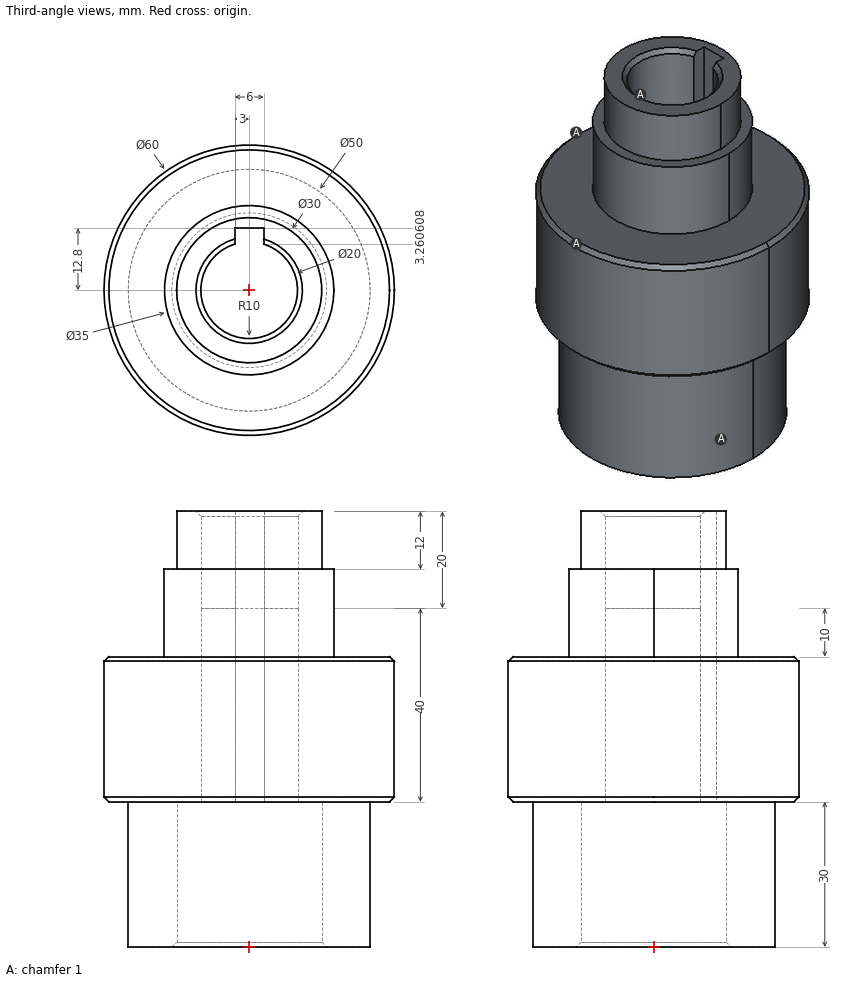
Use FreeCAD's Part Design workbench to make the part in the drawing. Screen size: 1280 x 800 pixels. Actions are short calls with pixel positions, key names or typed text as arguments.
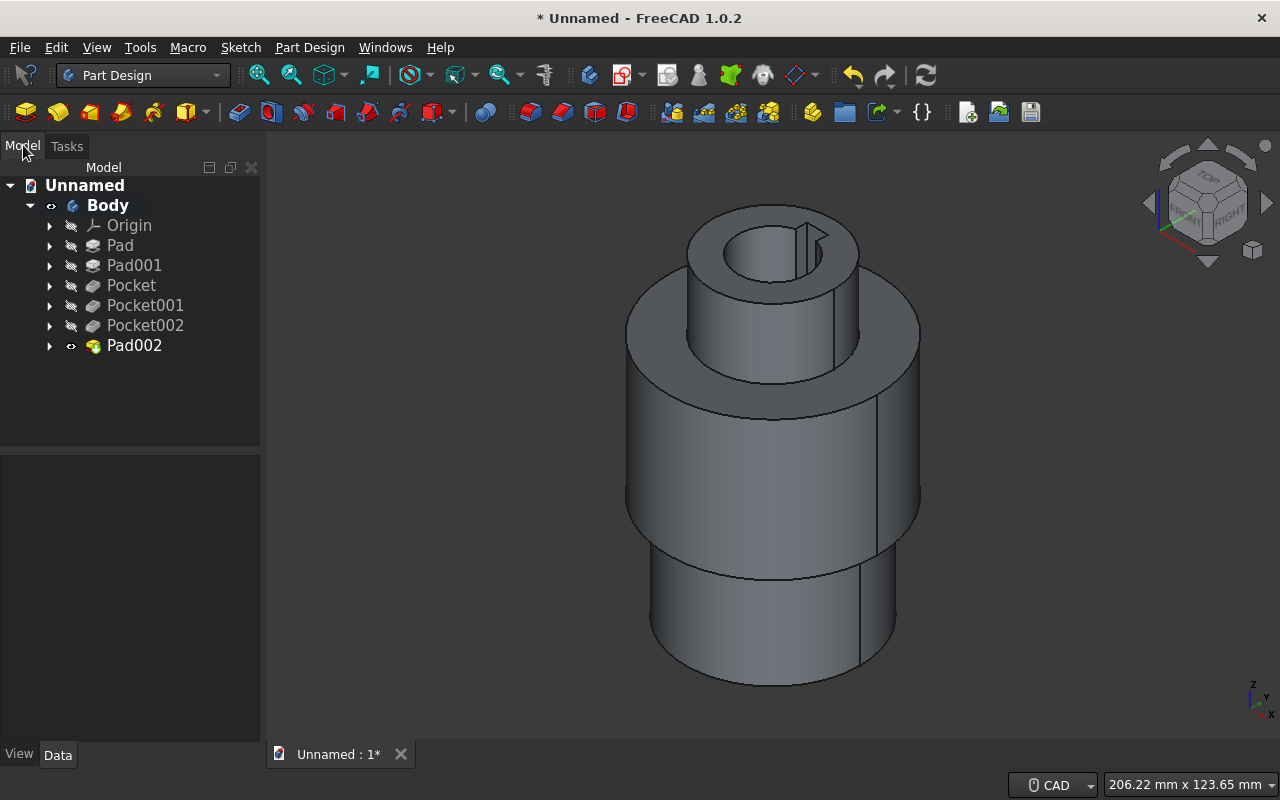
click(50, 226)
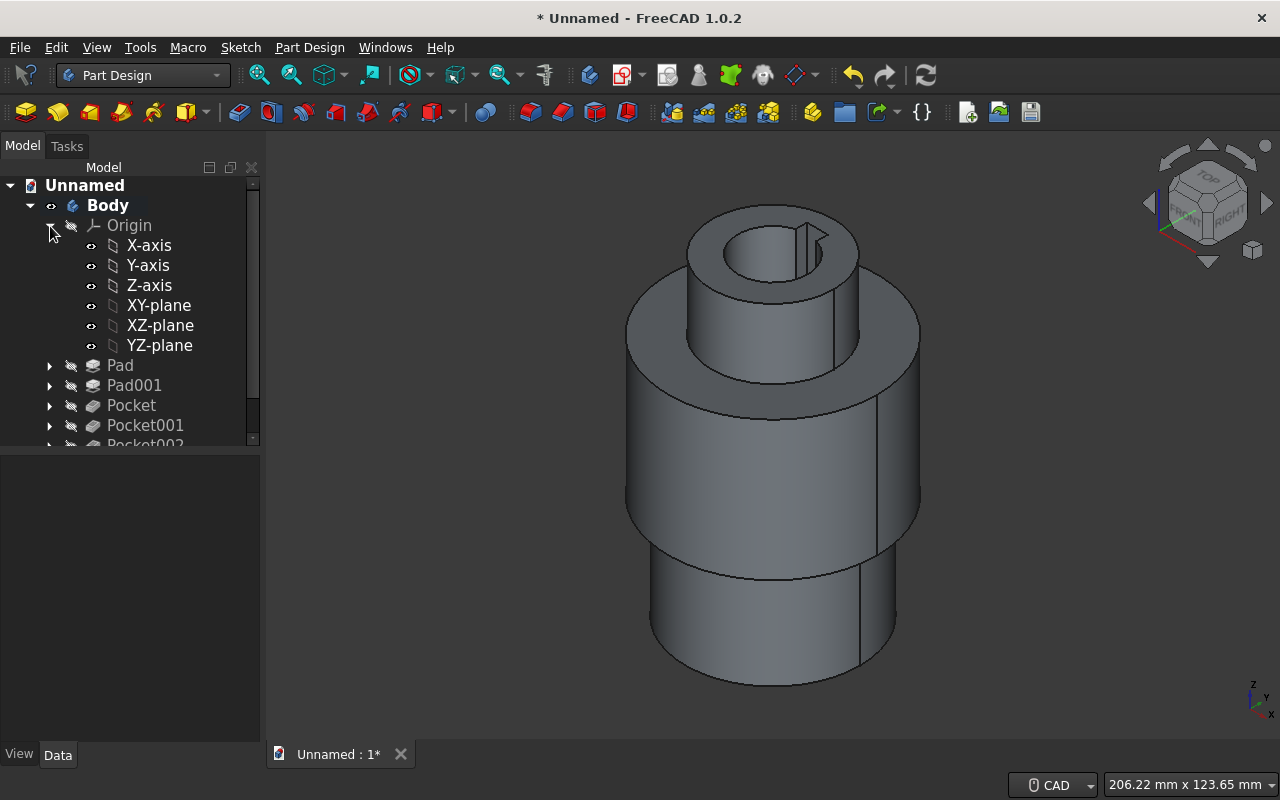
click(136, 306)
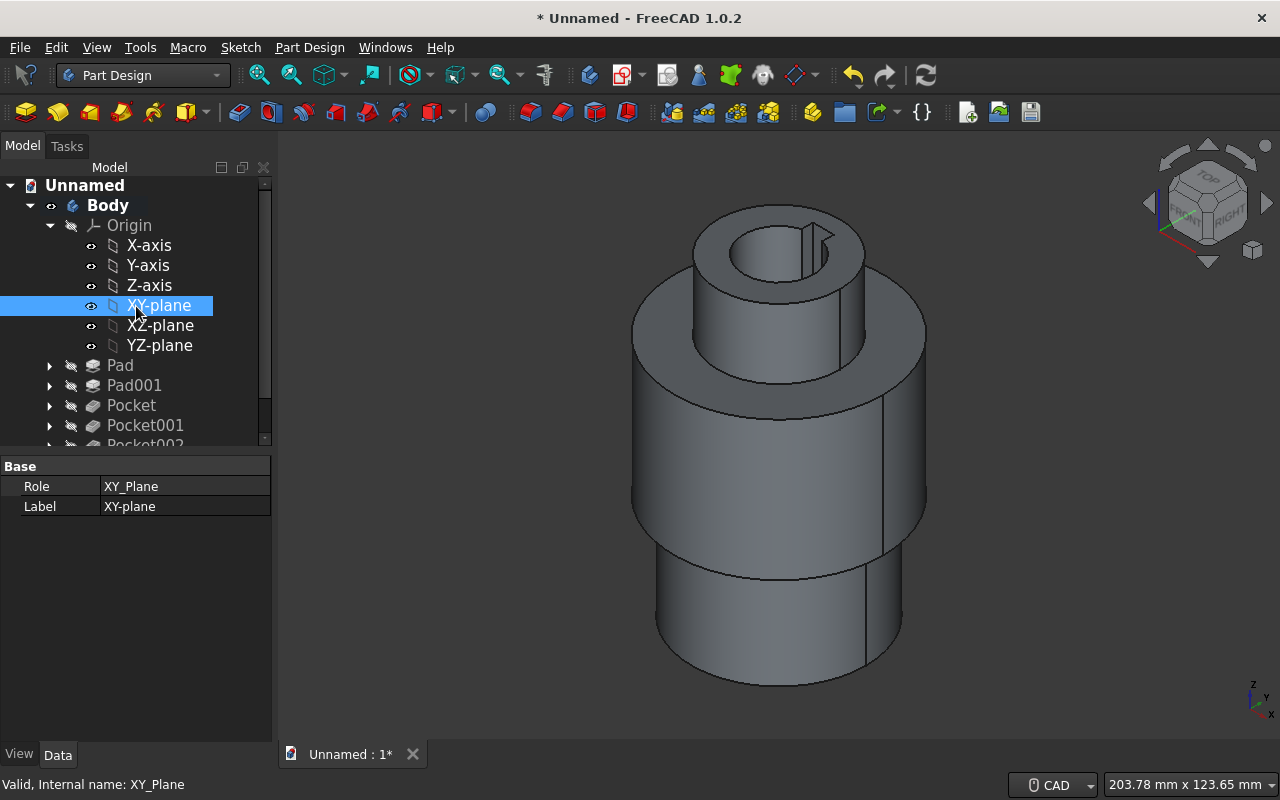
click(796, 76)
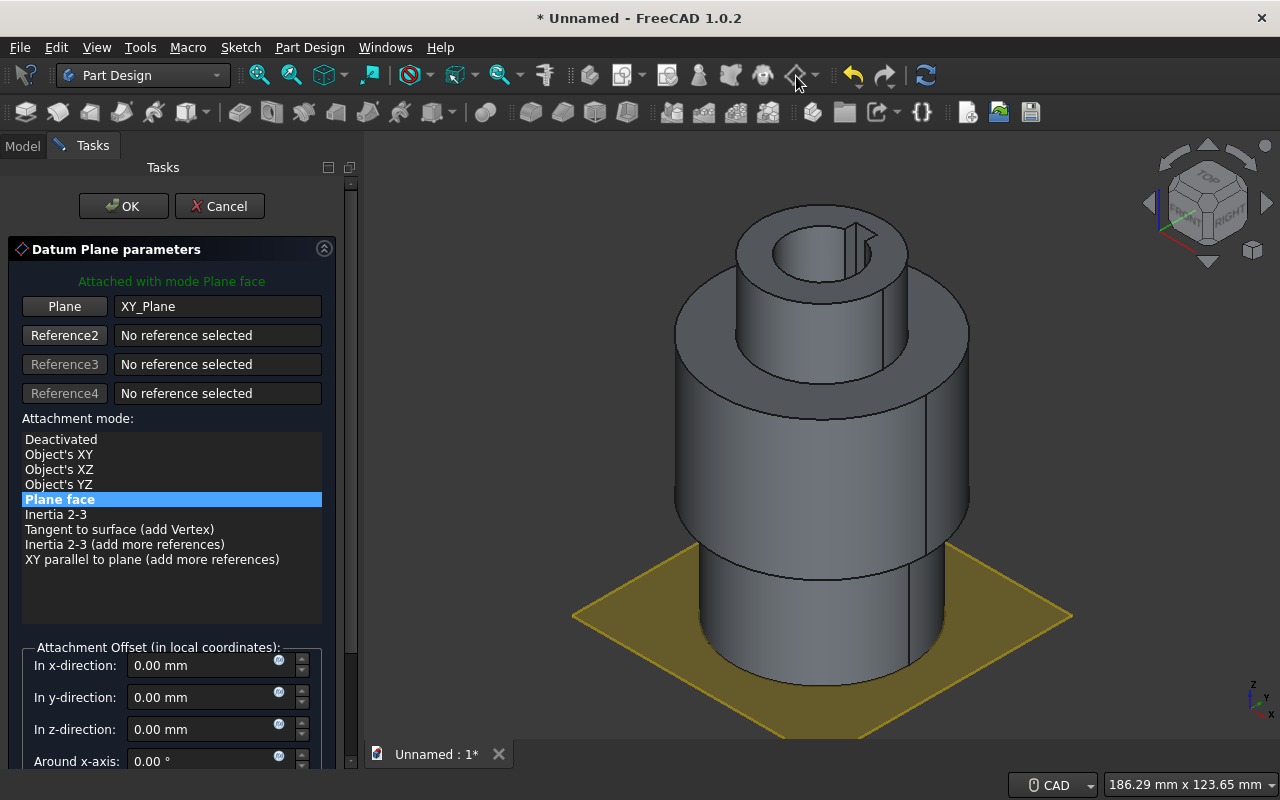
triple_click(210, 729)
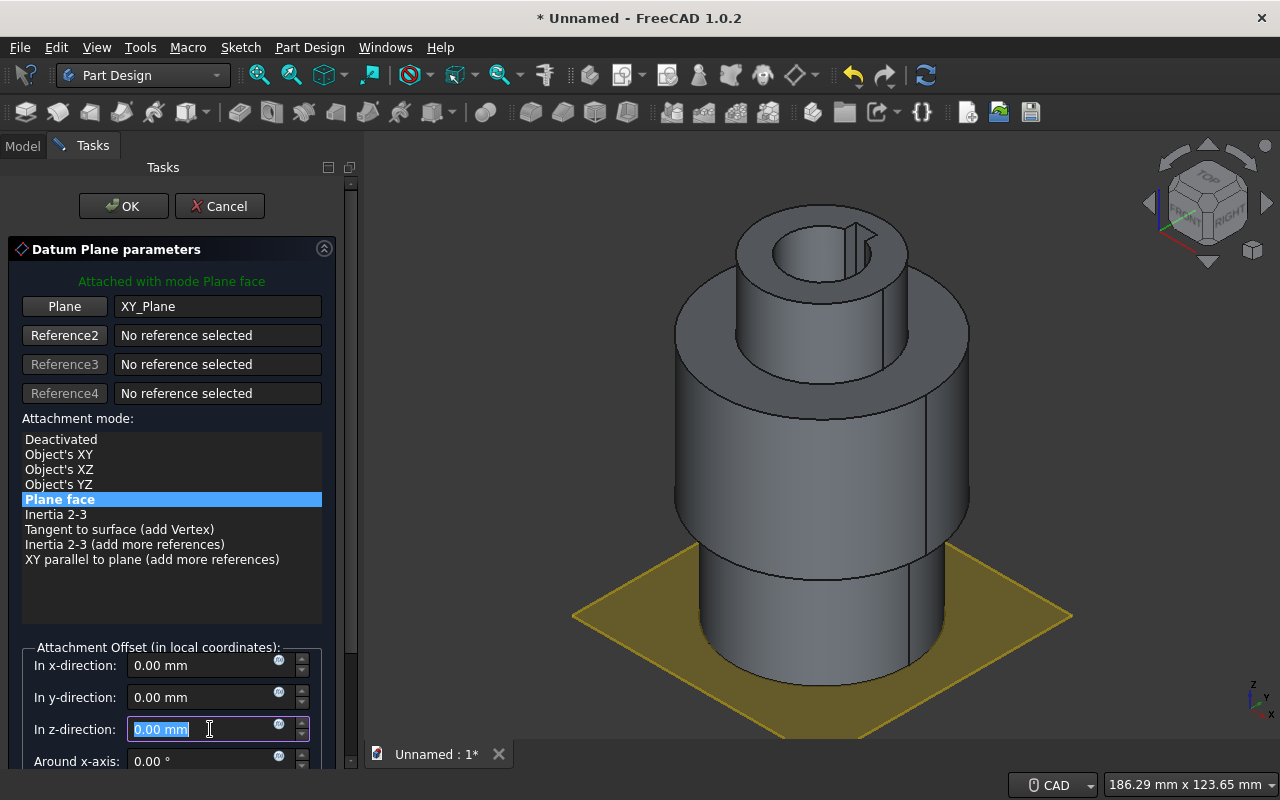
text(60)
key(Tab)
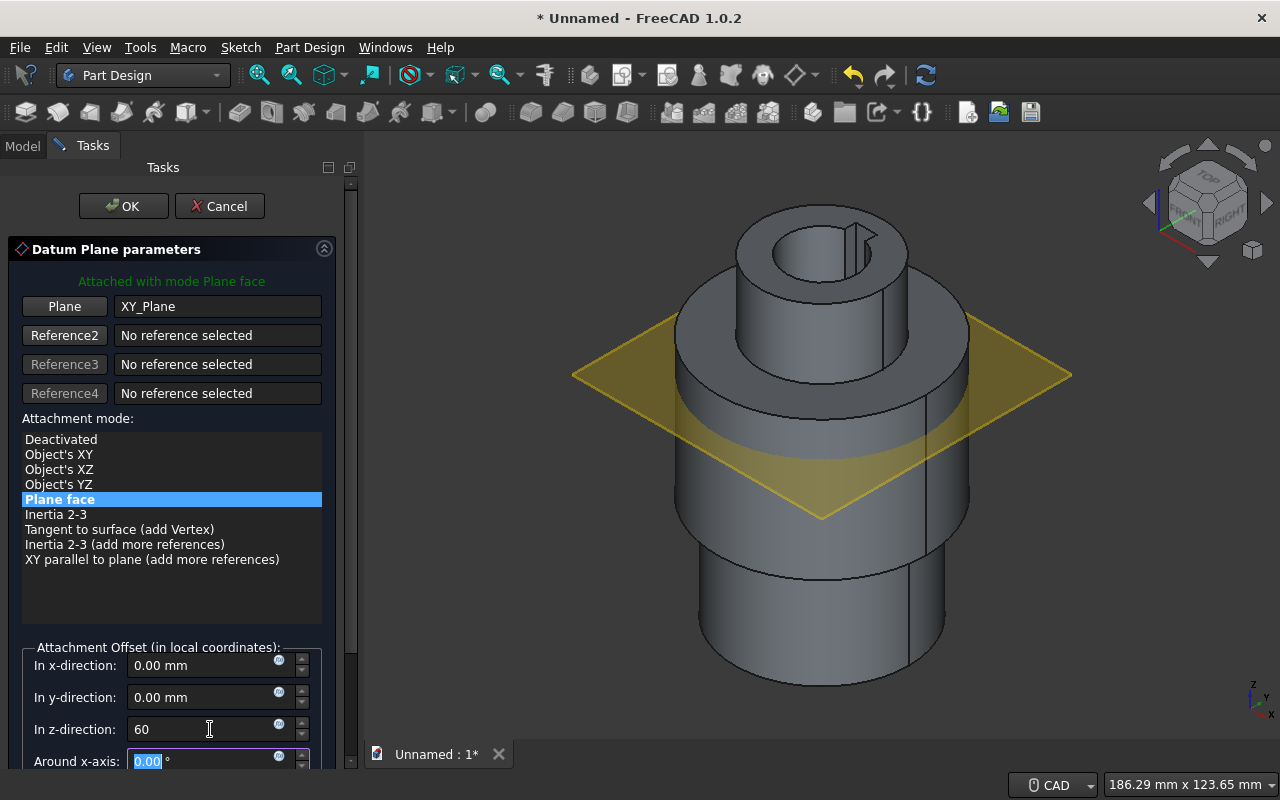
click(124, 206)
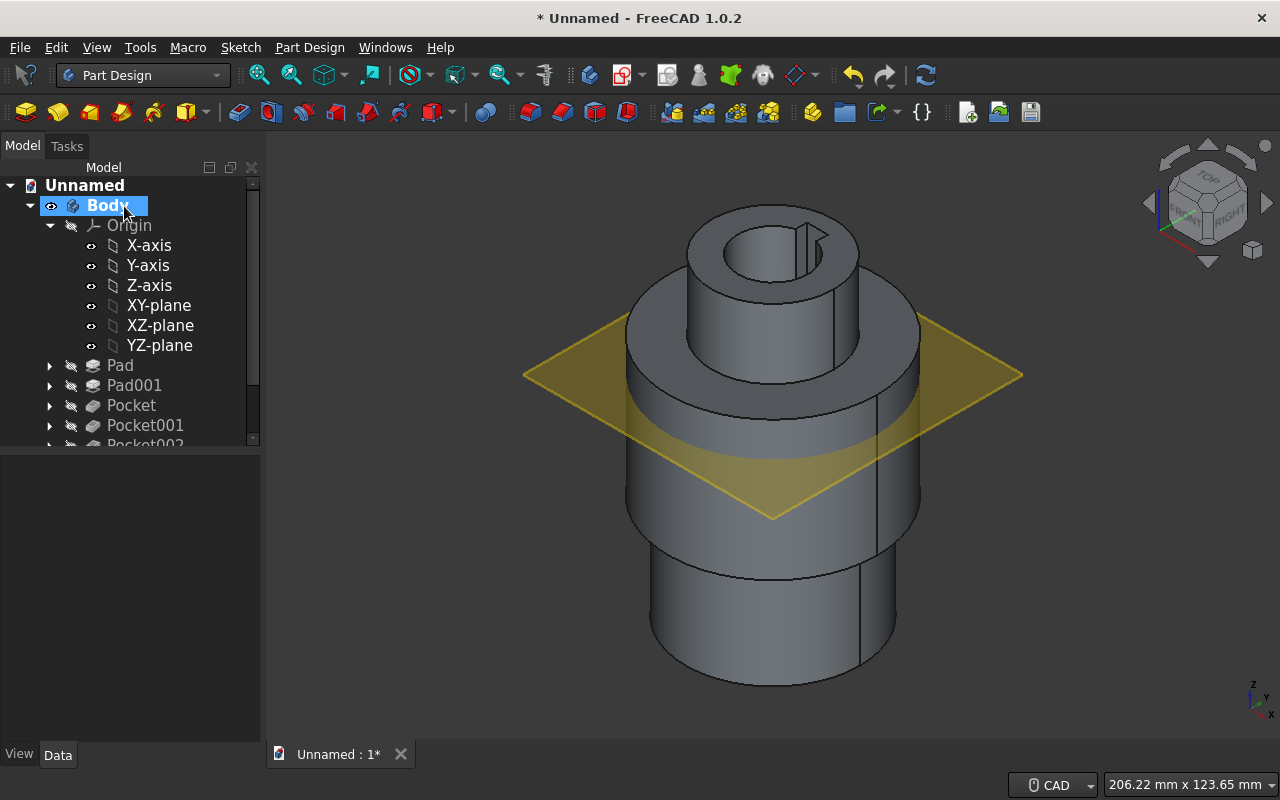
scroll(100, 321, down, 3)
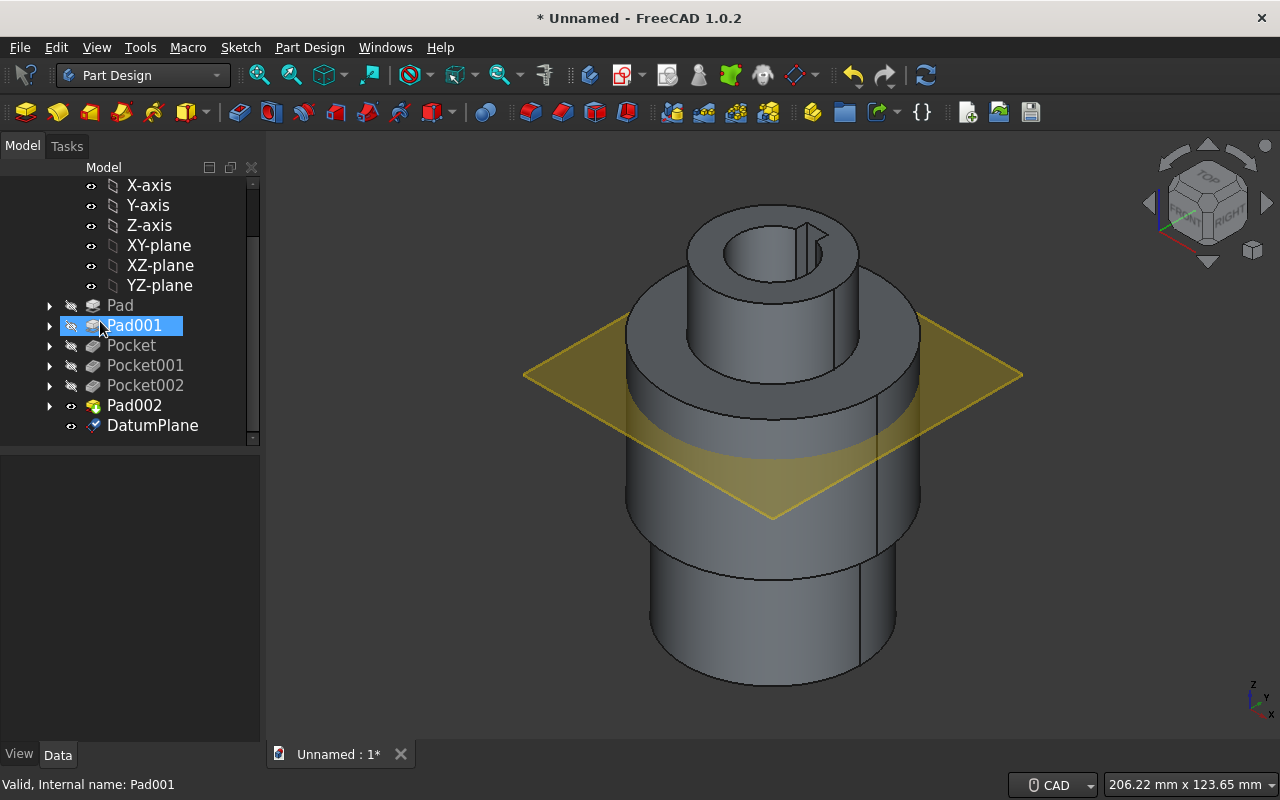
click(116, 426)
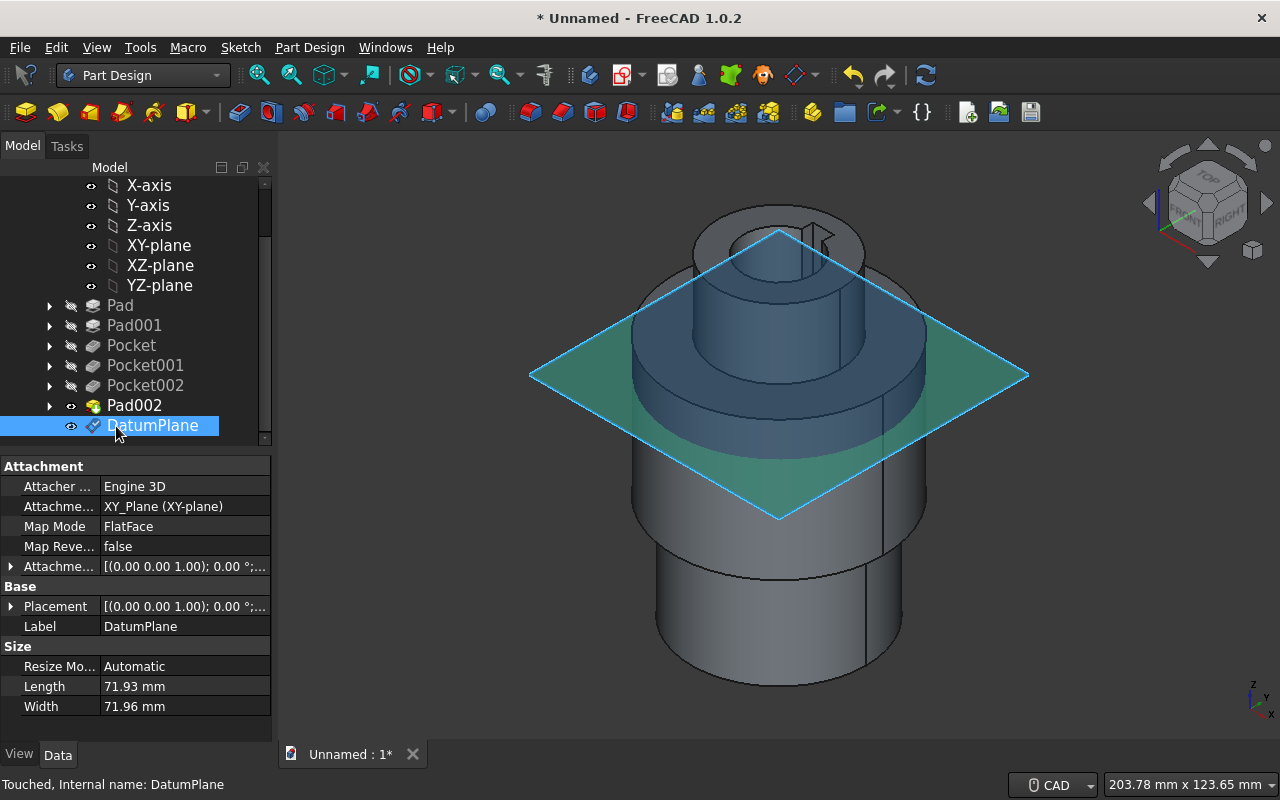
click(622, 76)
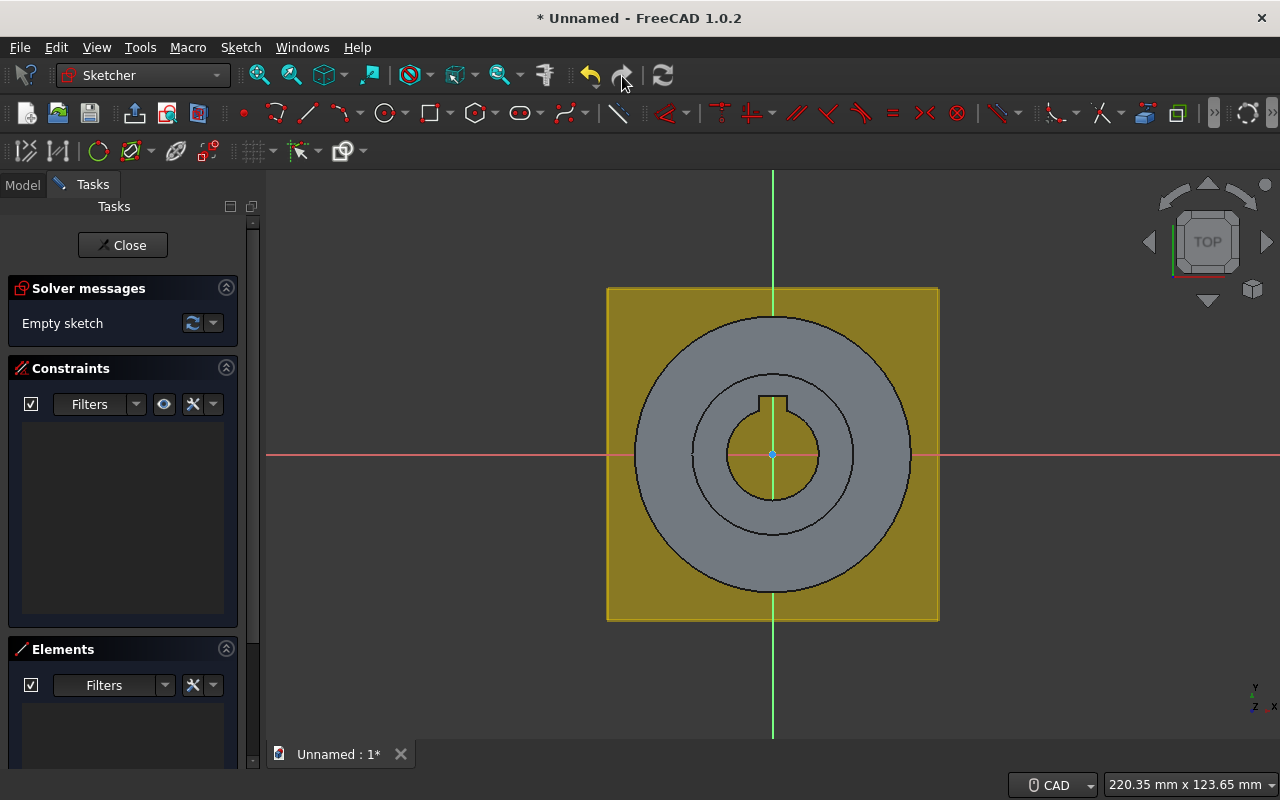
click(200, 114)